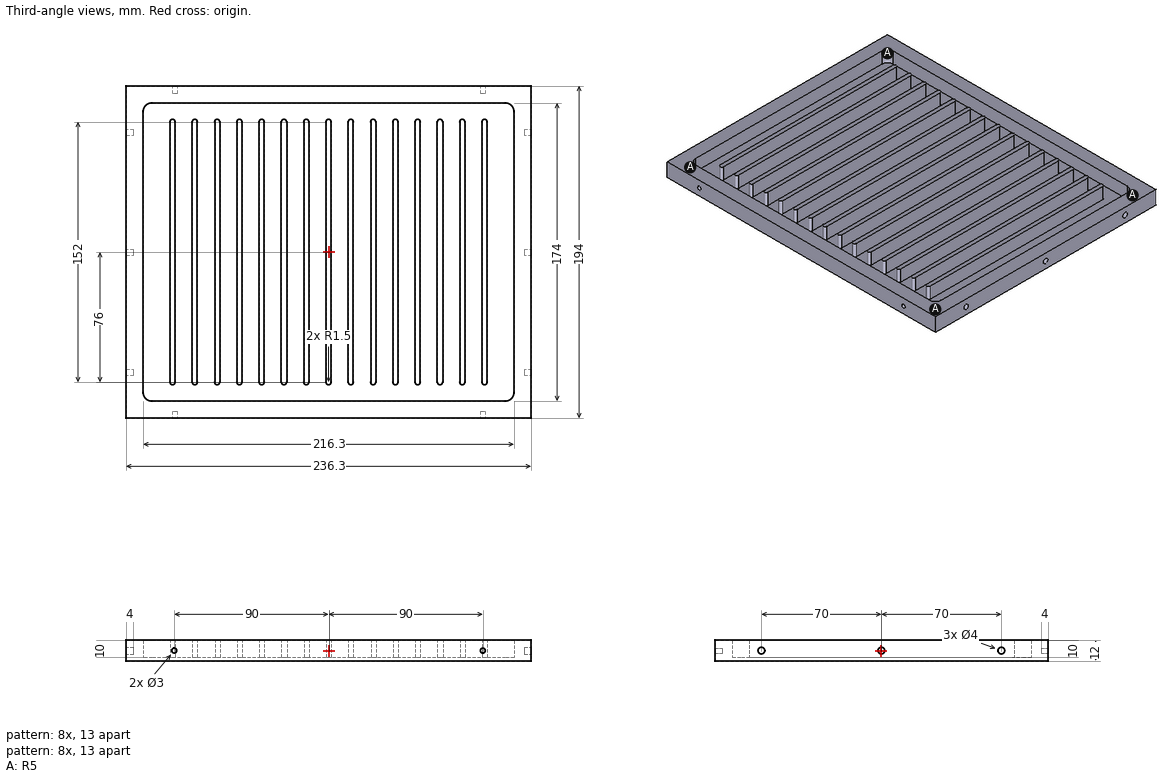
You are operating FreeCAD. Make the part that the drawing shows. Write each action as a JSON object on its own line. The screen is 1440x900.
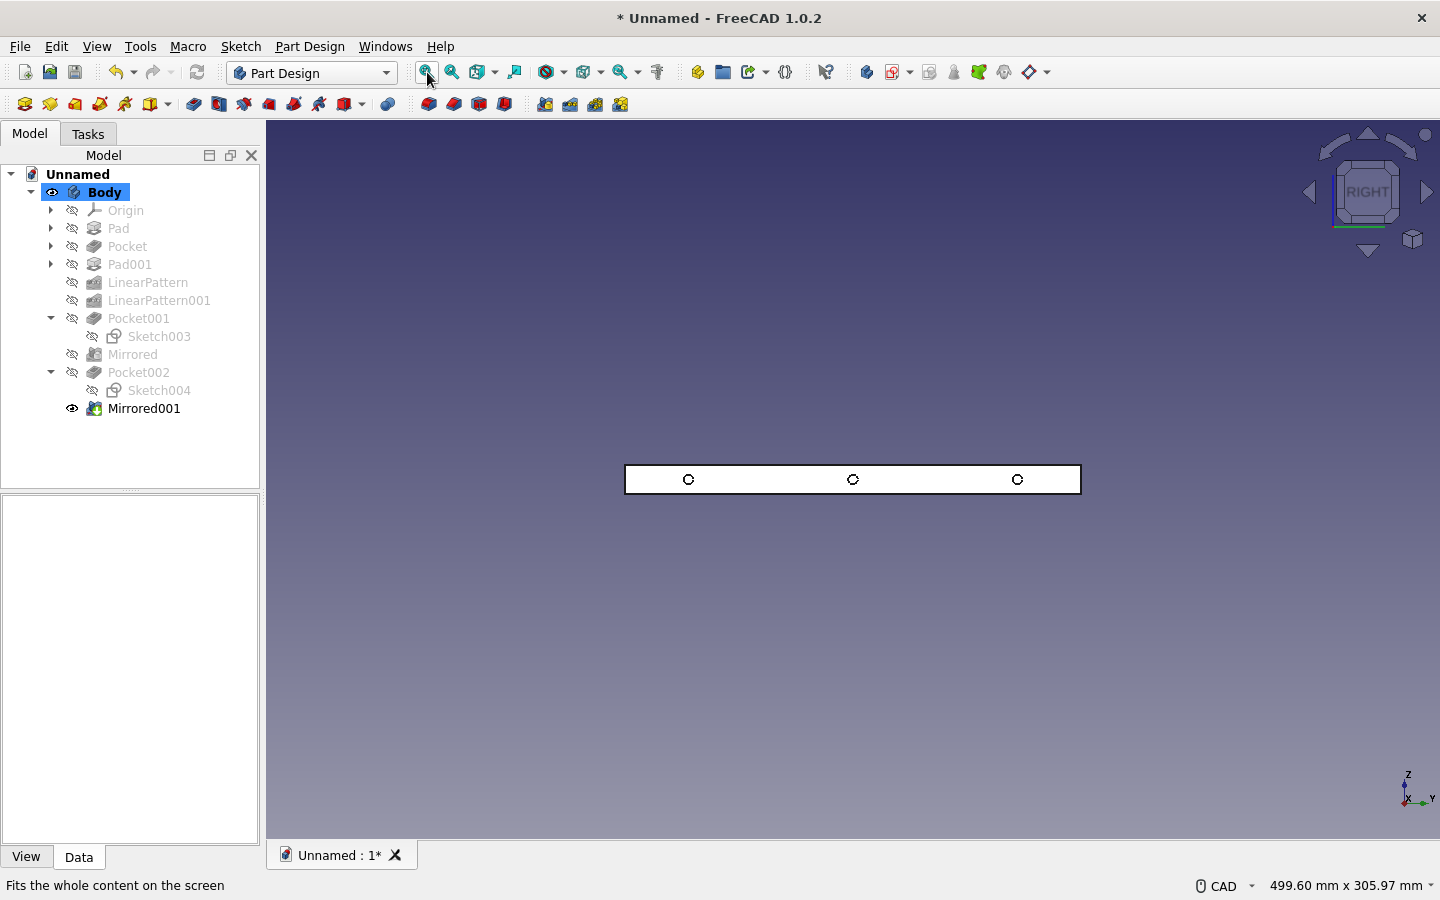
{"action": "key", "text": "5"}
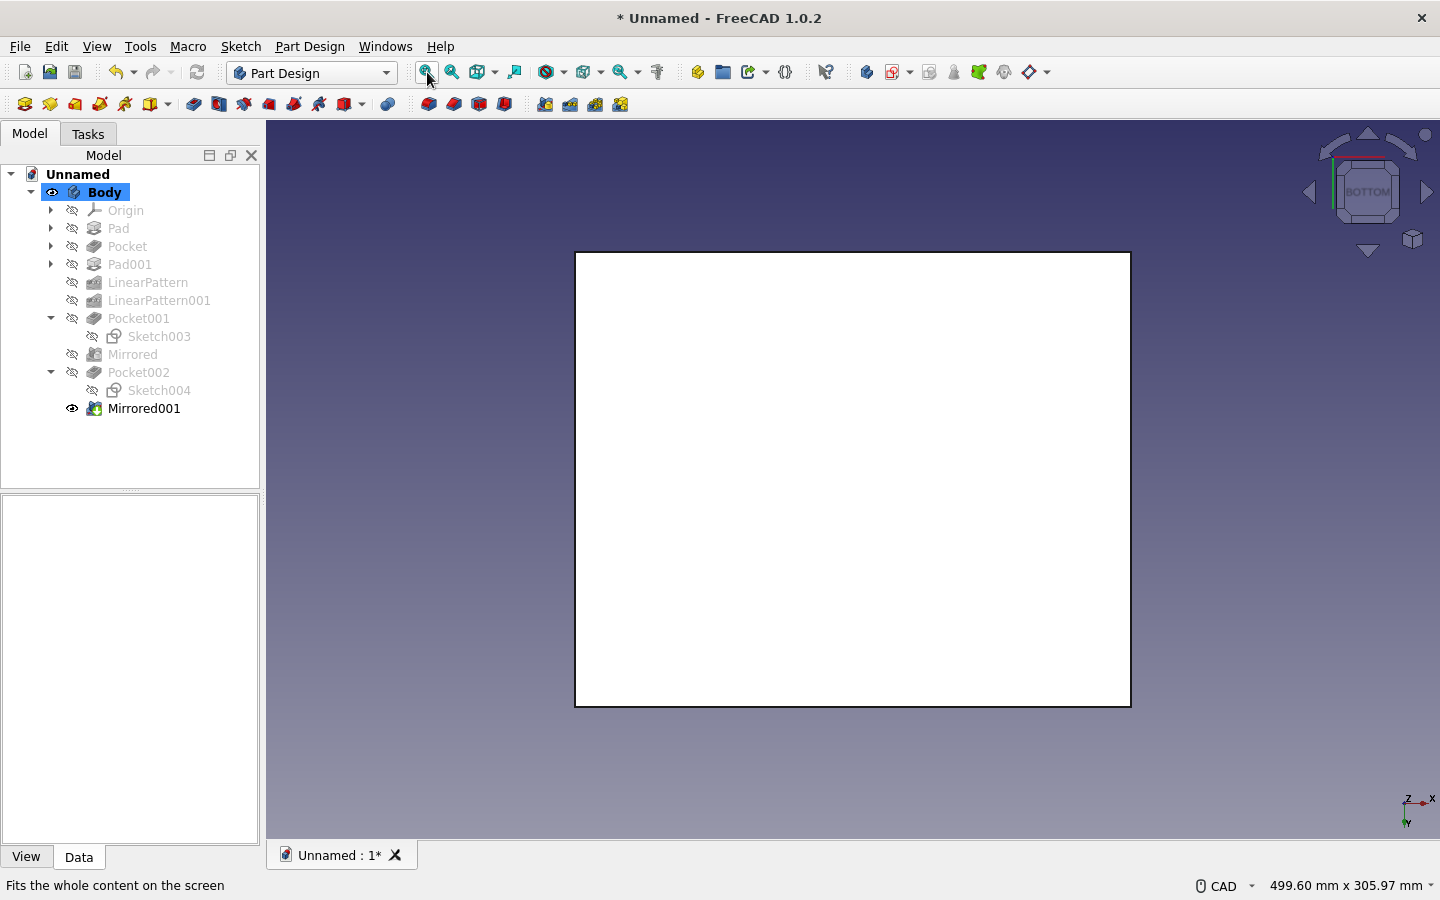
{"action": "key", "text": "4"}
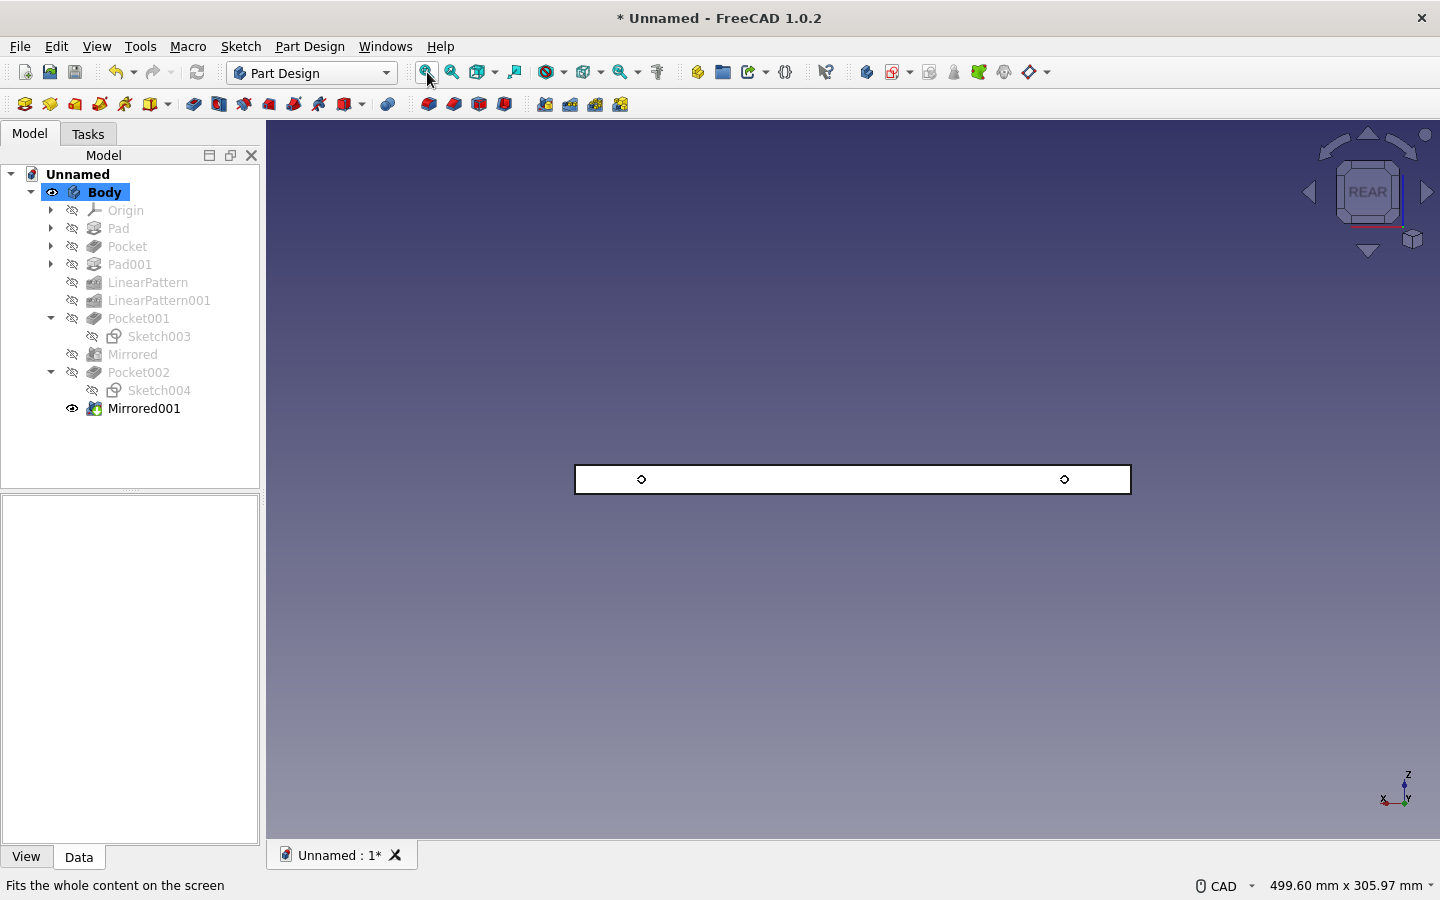
{"action": "key", "text": "6"}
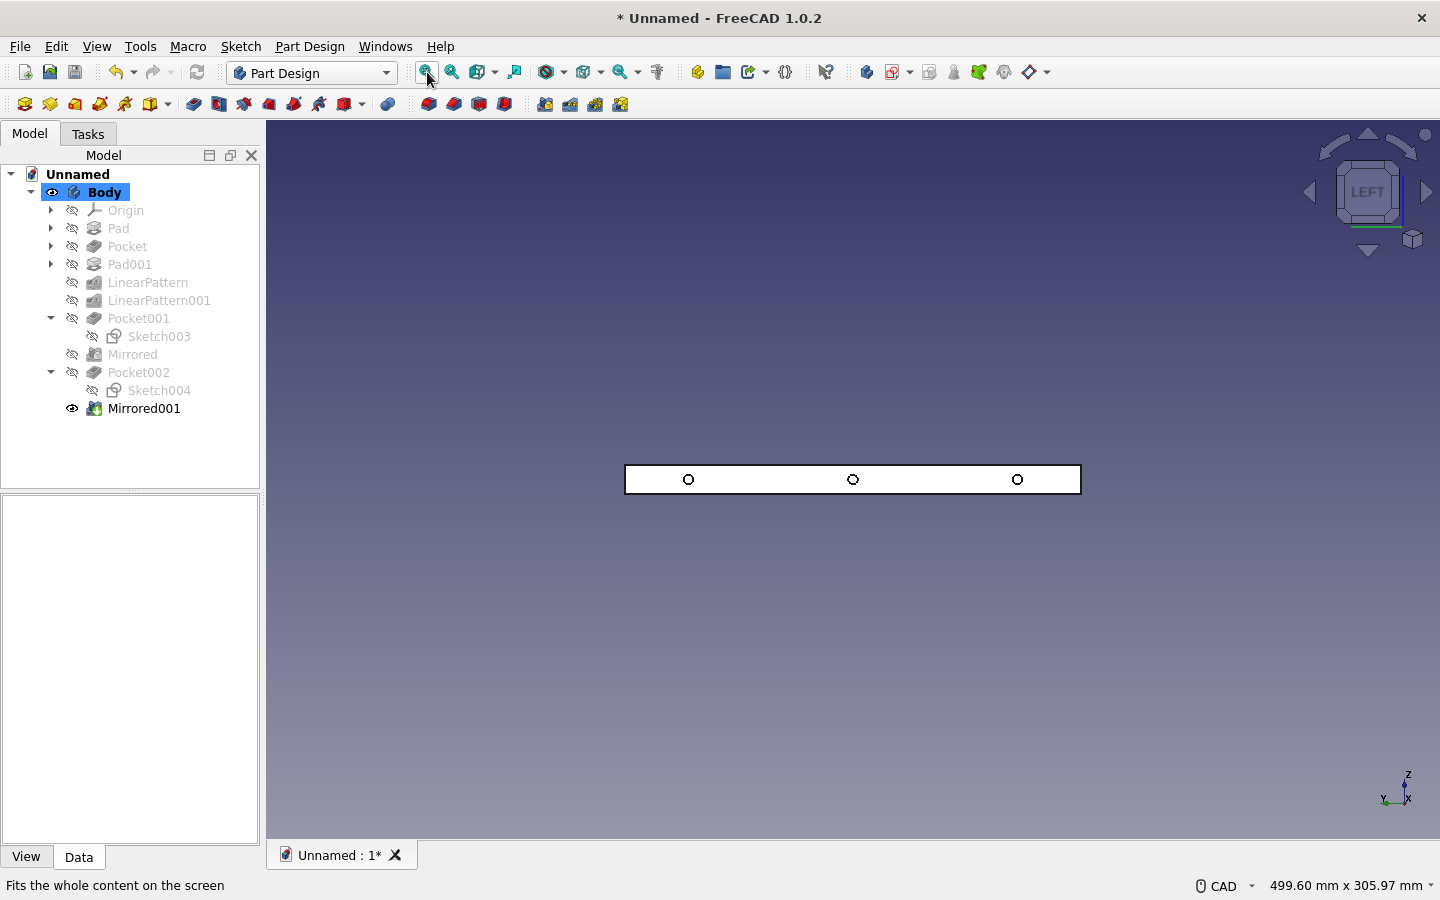
{"action": "left_click", "coordinate": [427, 72]}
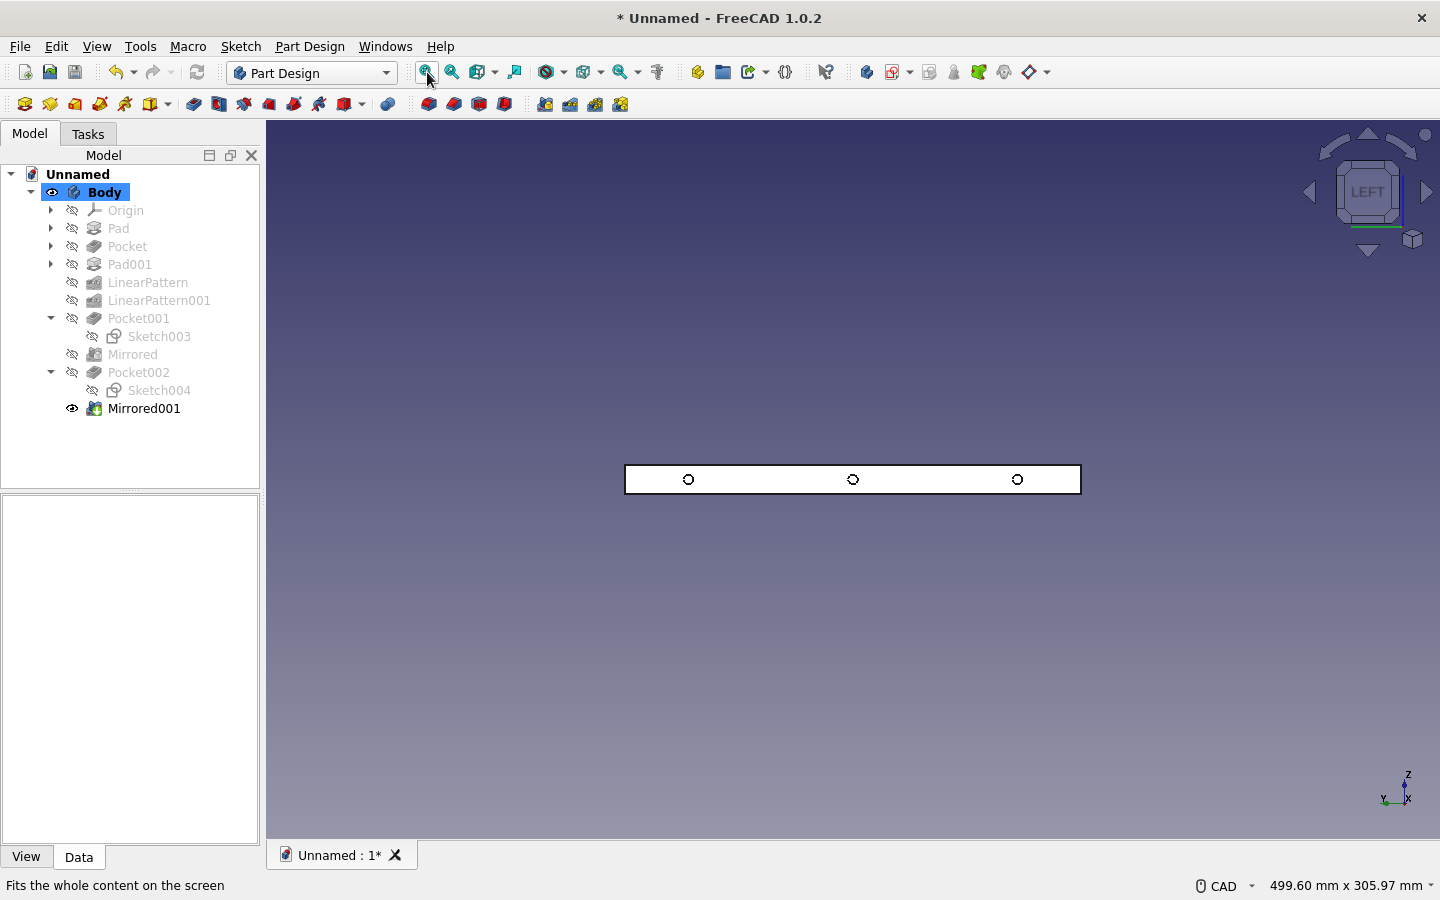
{"action": "key", "text": "v 3"}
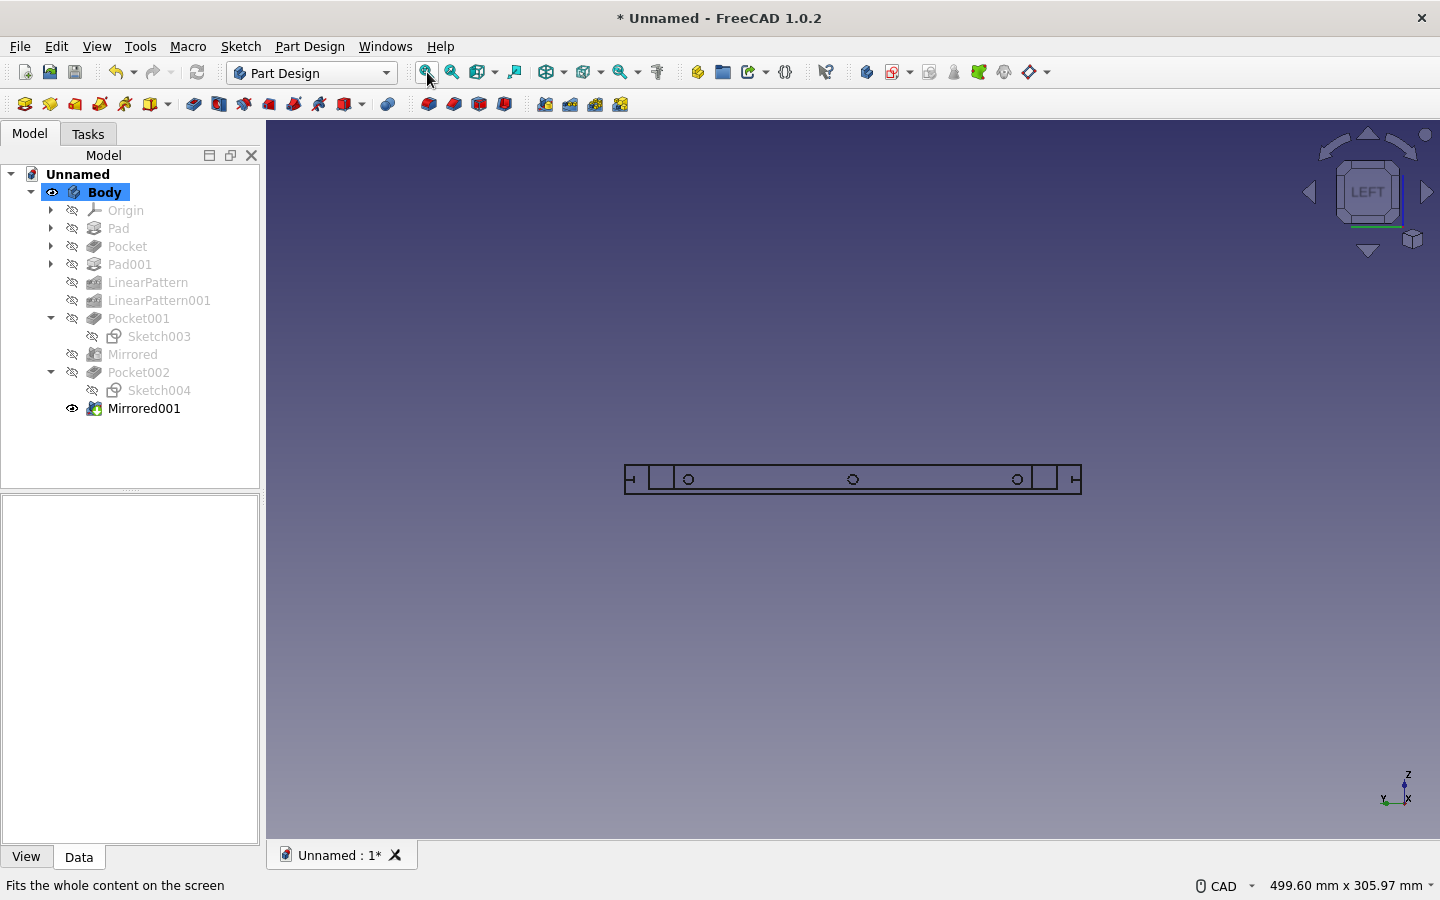
{"action": "key", "text": "0"}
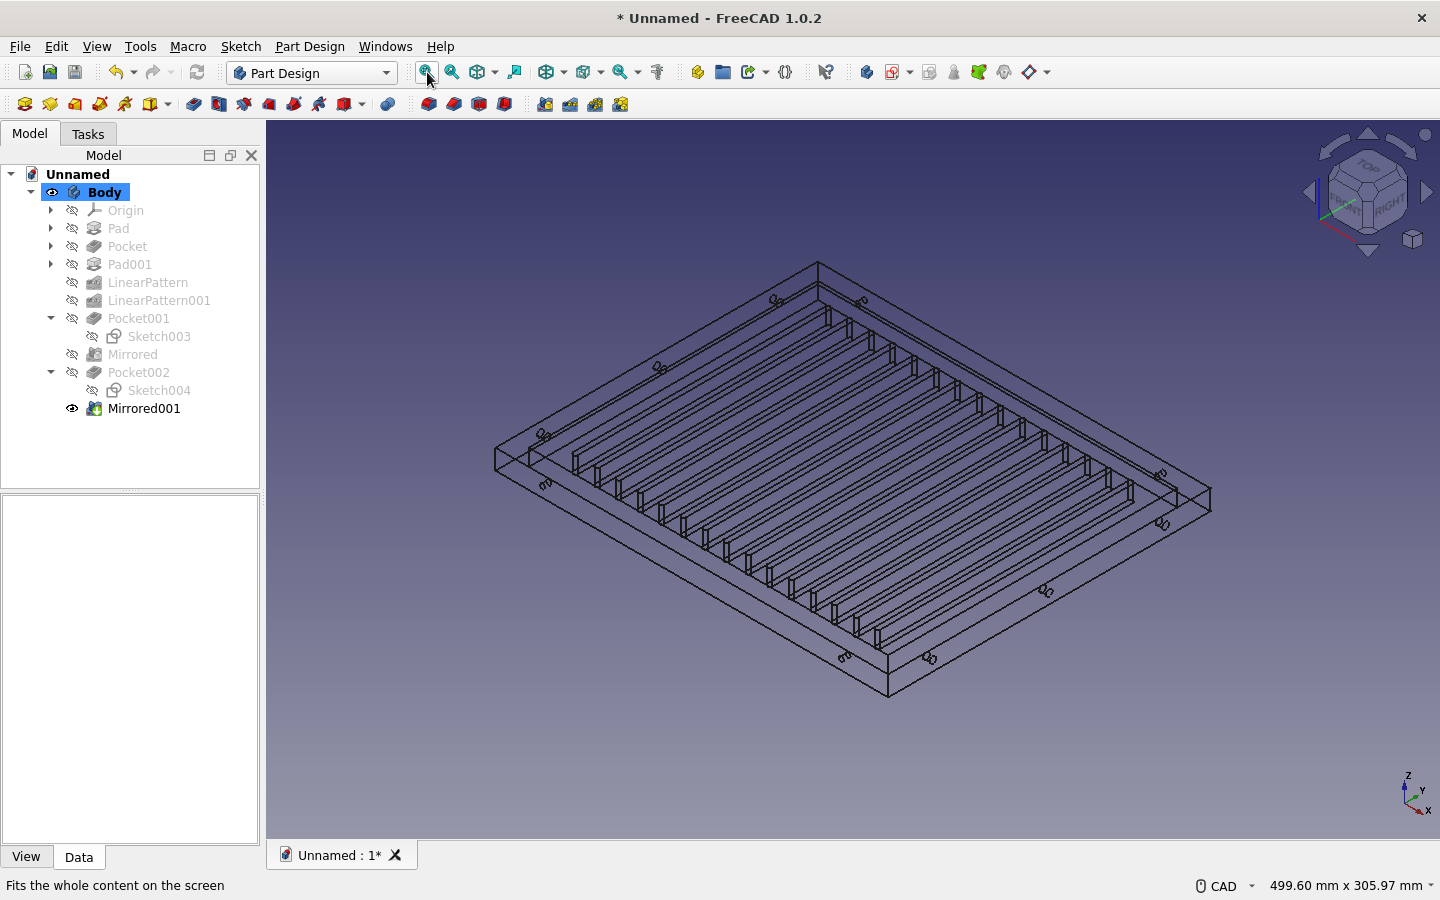
{"action": "left_click", "coordinate": [818, 289]}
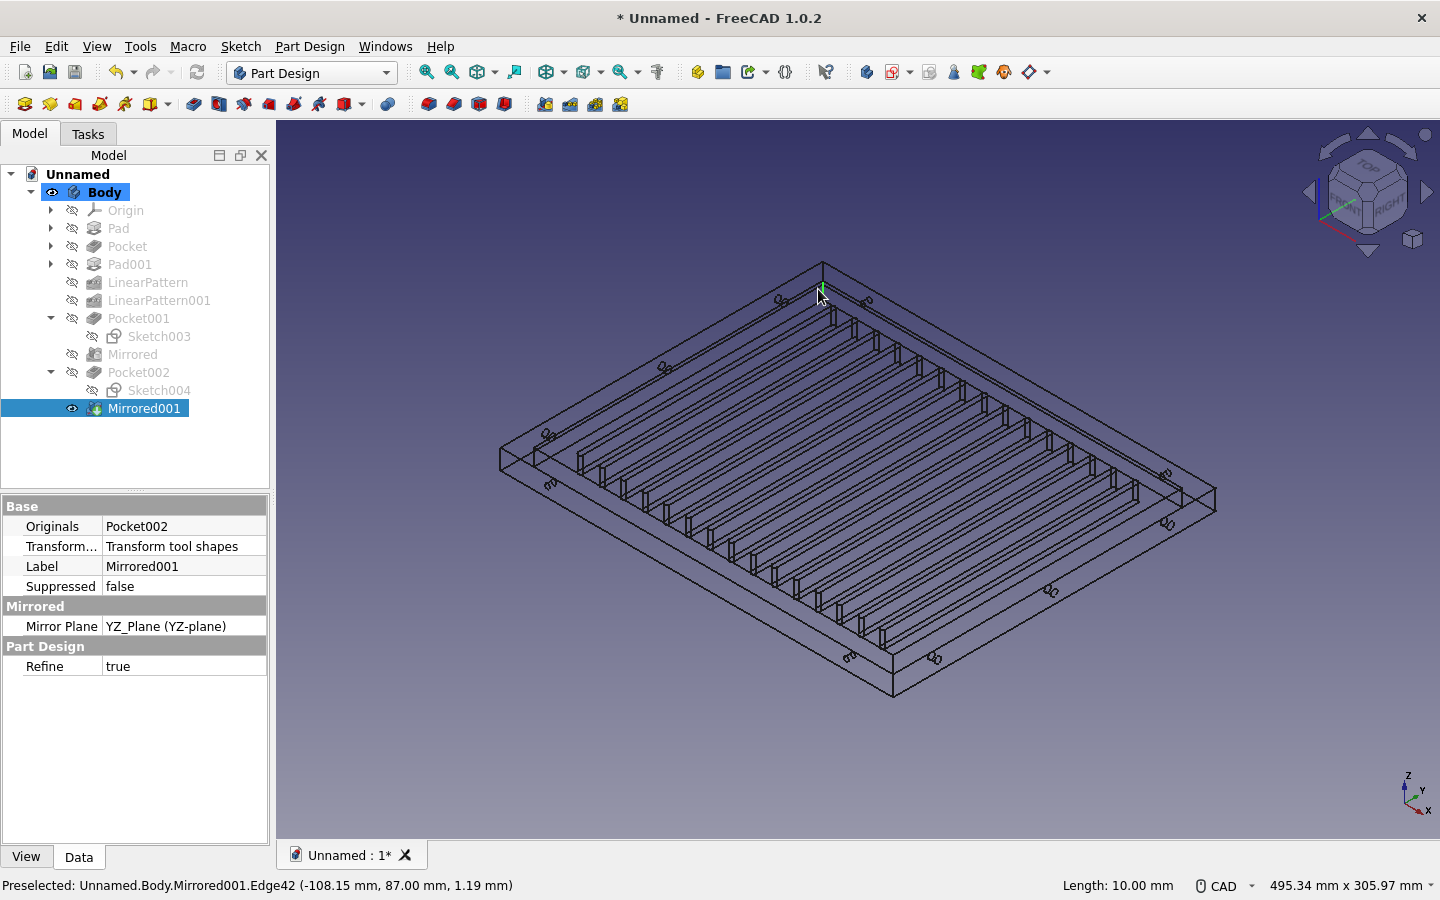
{"action": "left_click", "coordinate": [1182, 497], "text": "ctrl"}